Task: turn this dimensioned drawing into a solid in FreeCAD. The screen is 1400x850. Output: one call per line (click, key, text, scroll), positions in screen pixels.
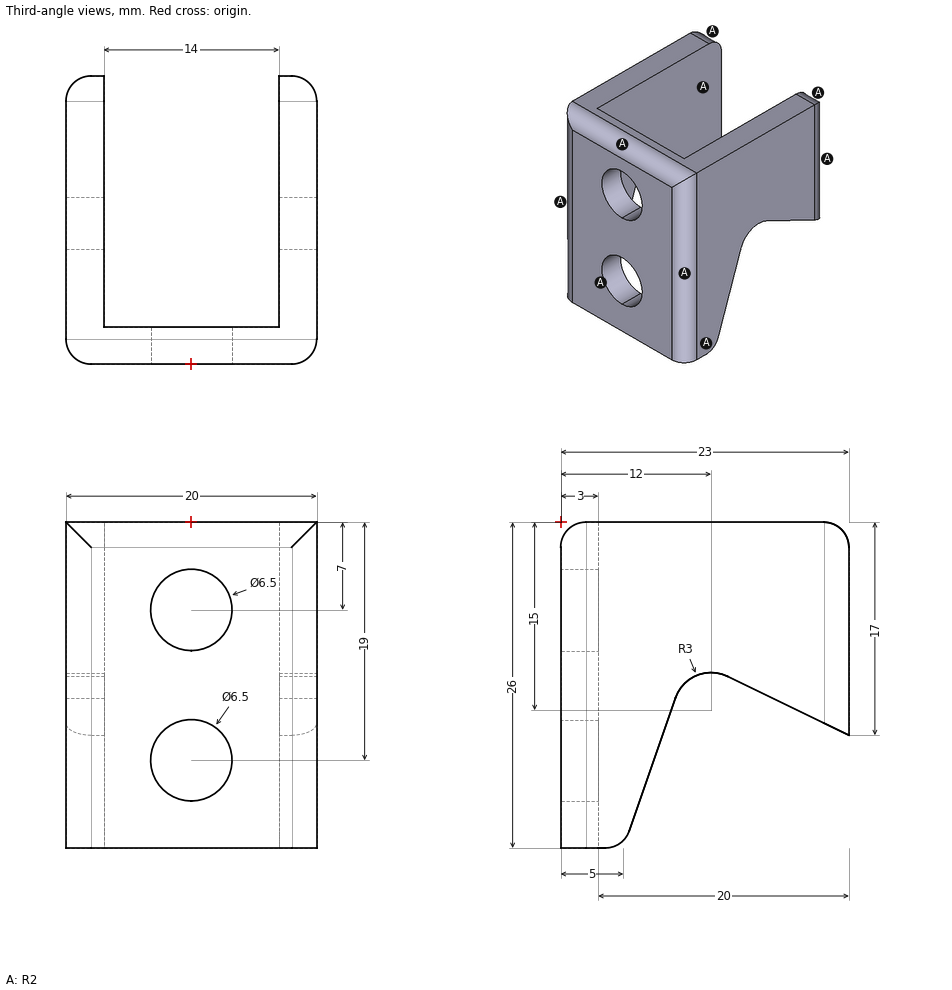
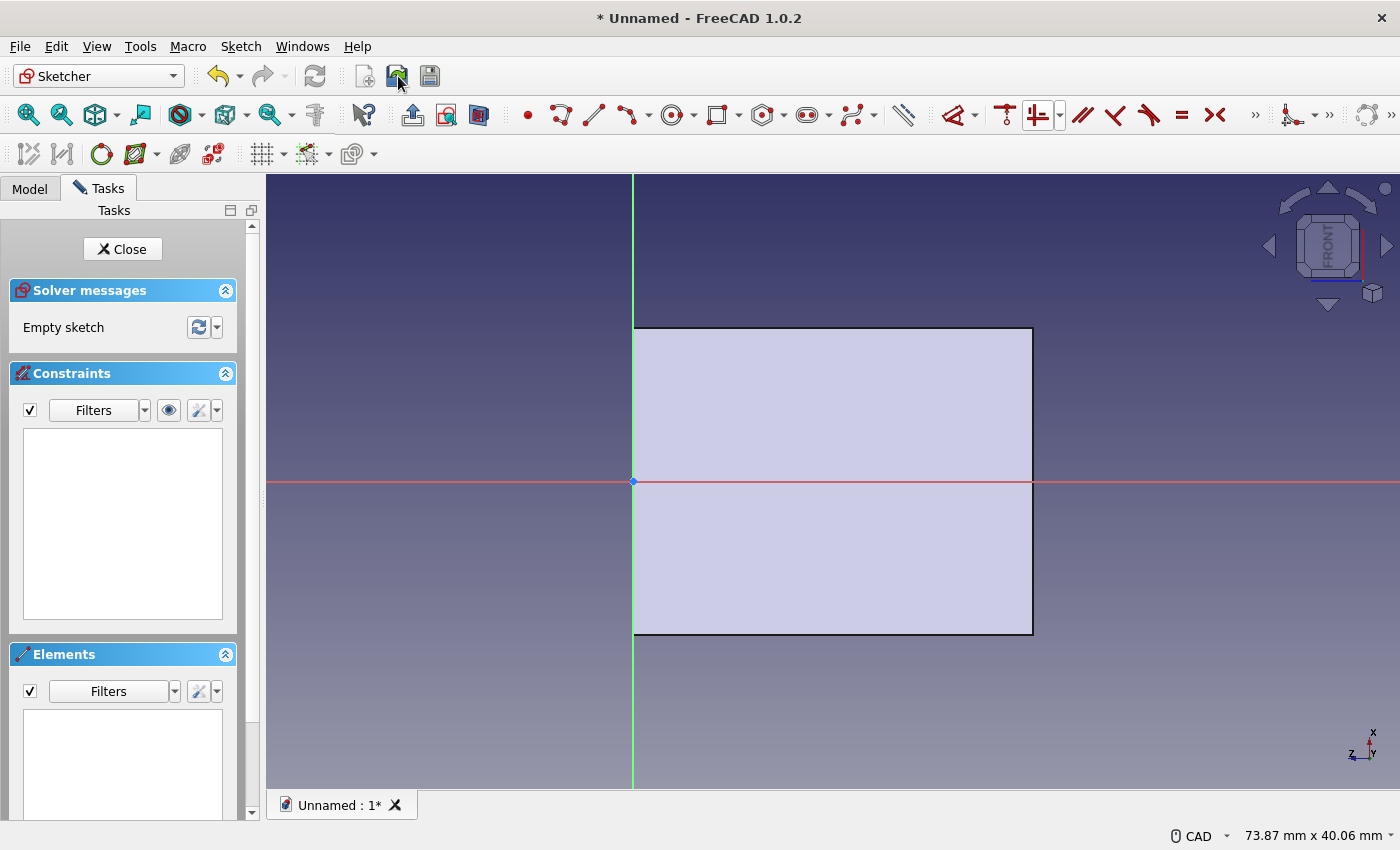
scroll(695, 481, up, 7)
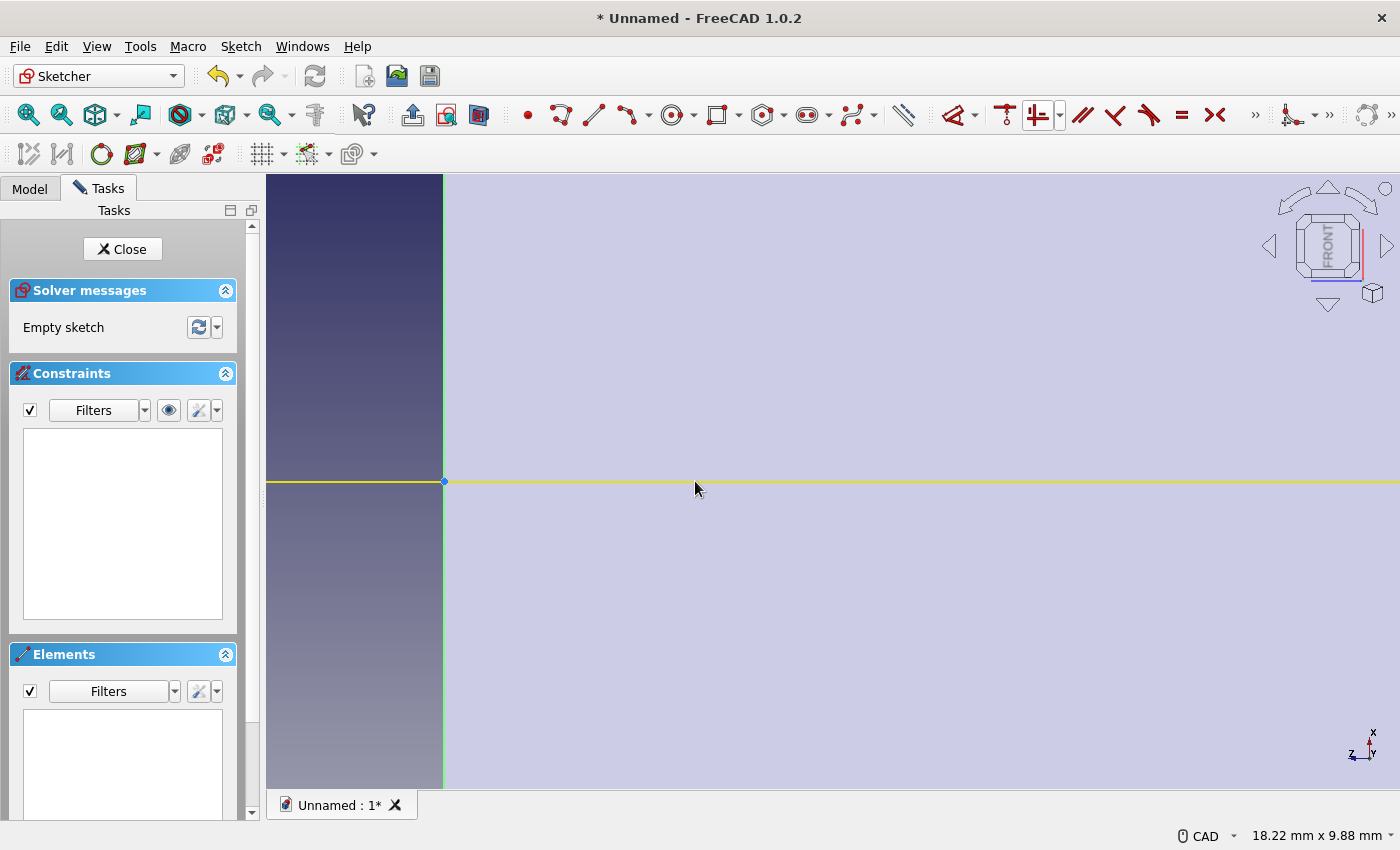
click(672, 116)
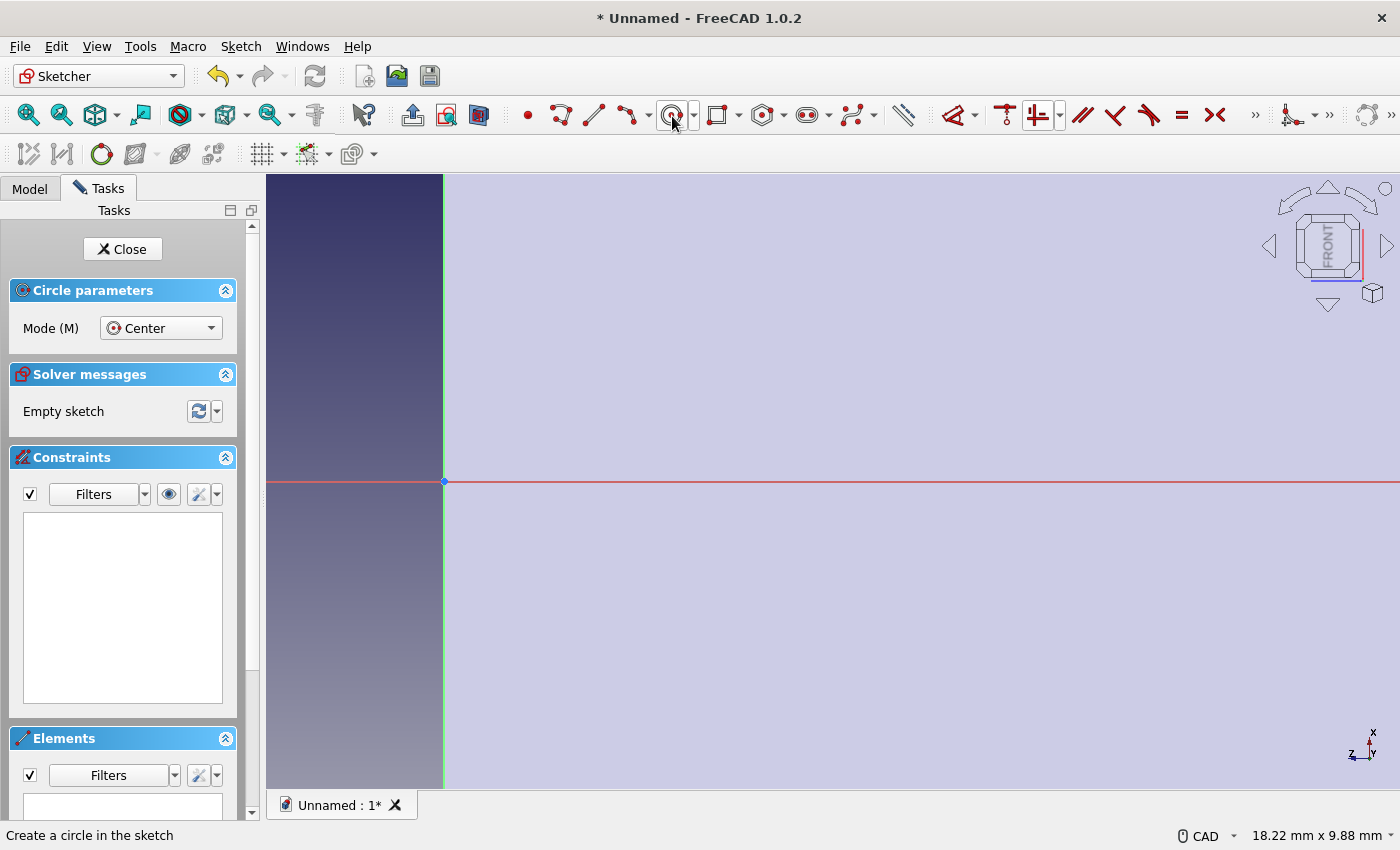
click(880, 482)
click(1023, 338)
key(Escape)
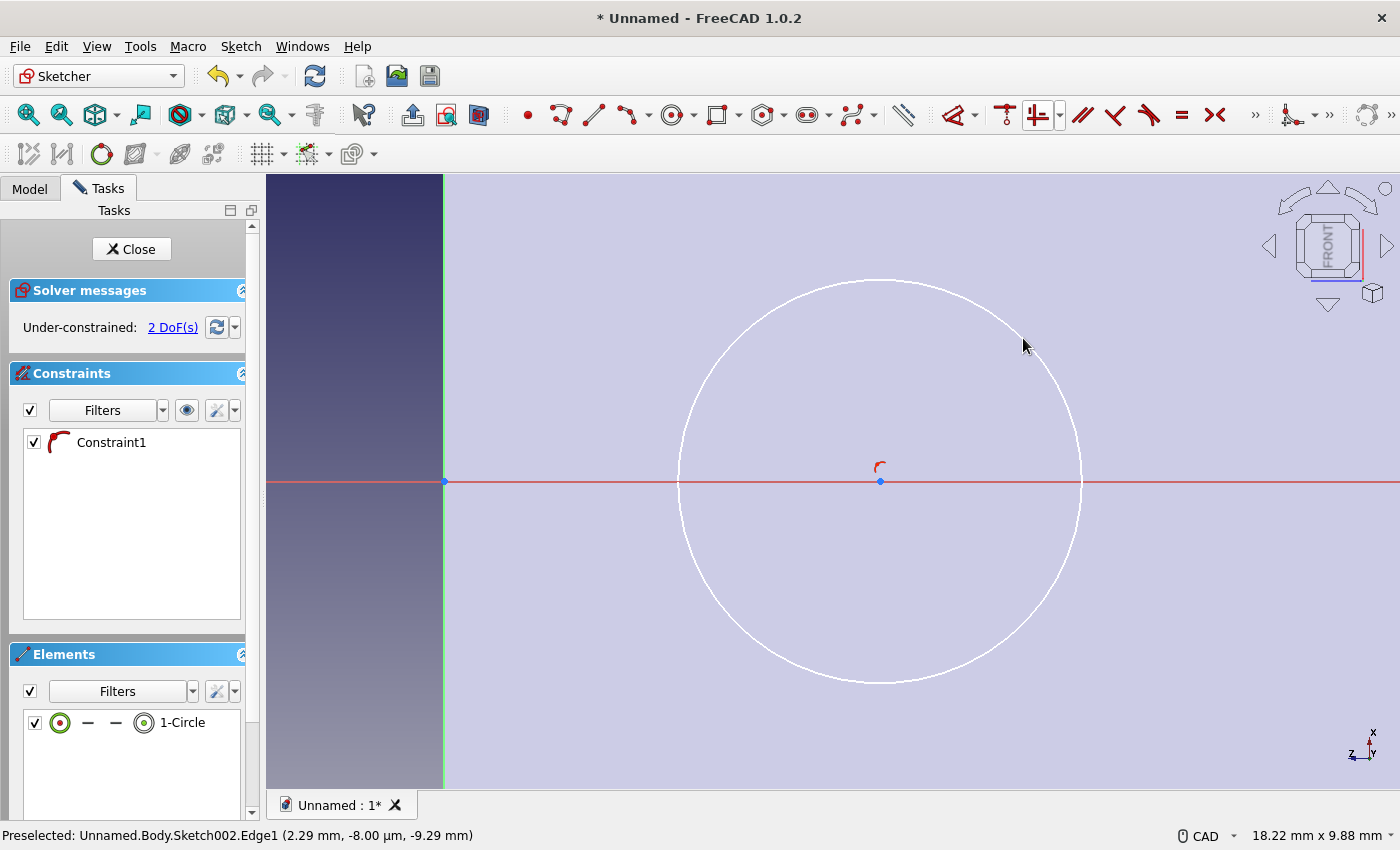
click(952, 116)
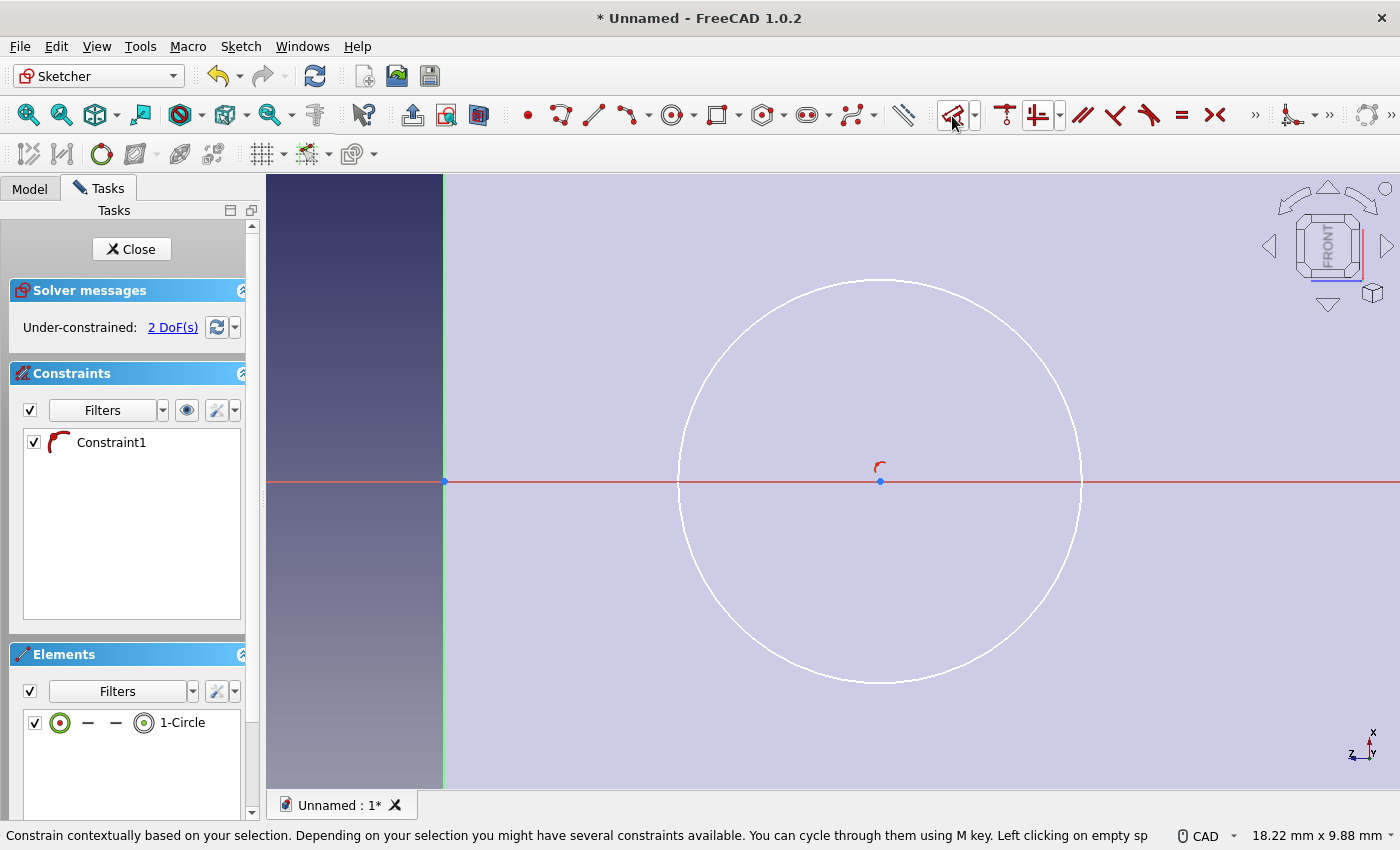
click(1022, 338)
click(1045, 315)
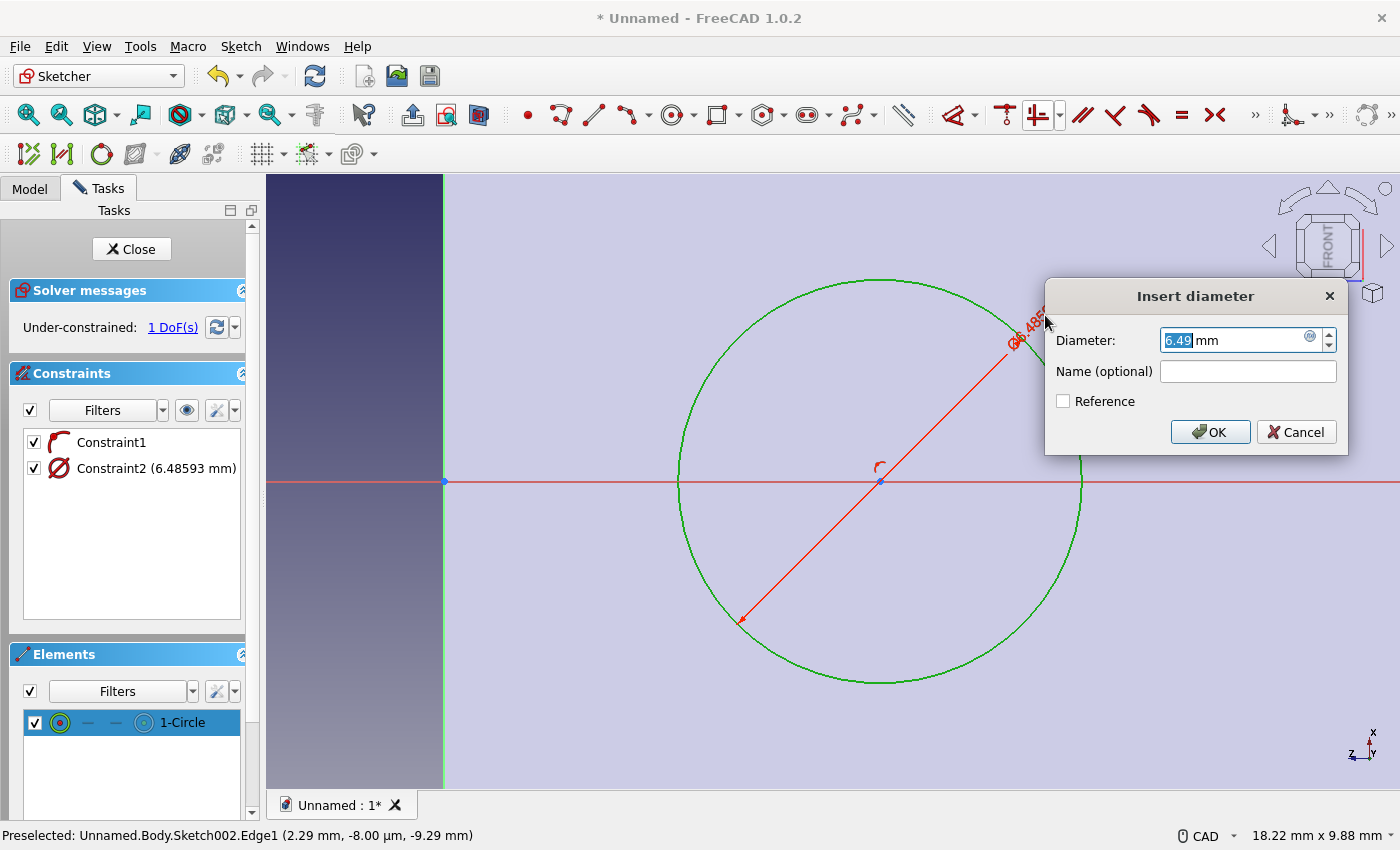
text(6.5)
key(Return)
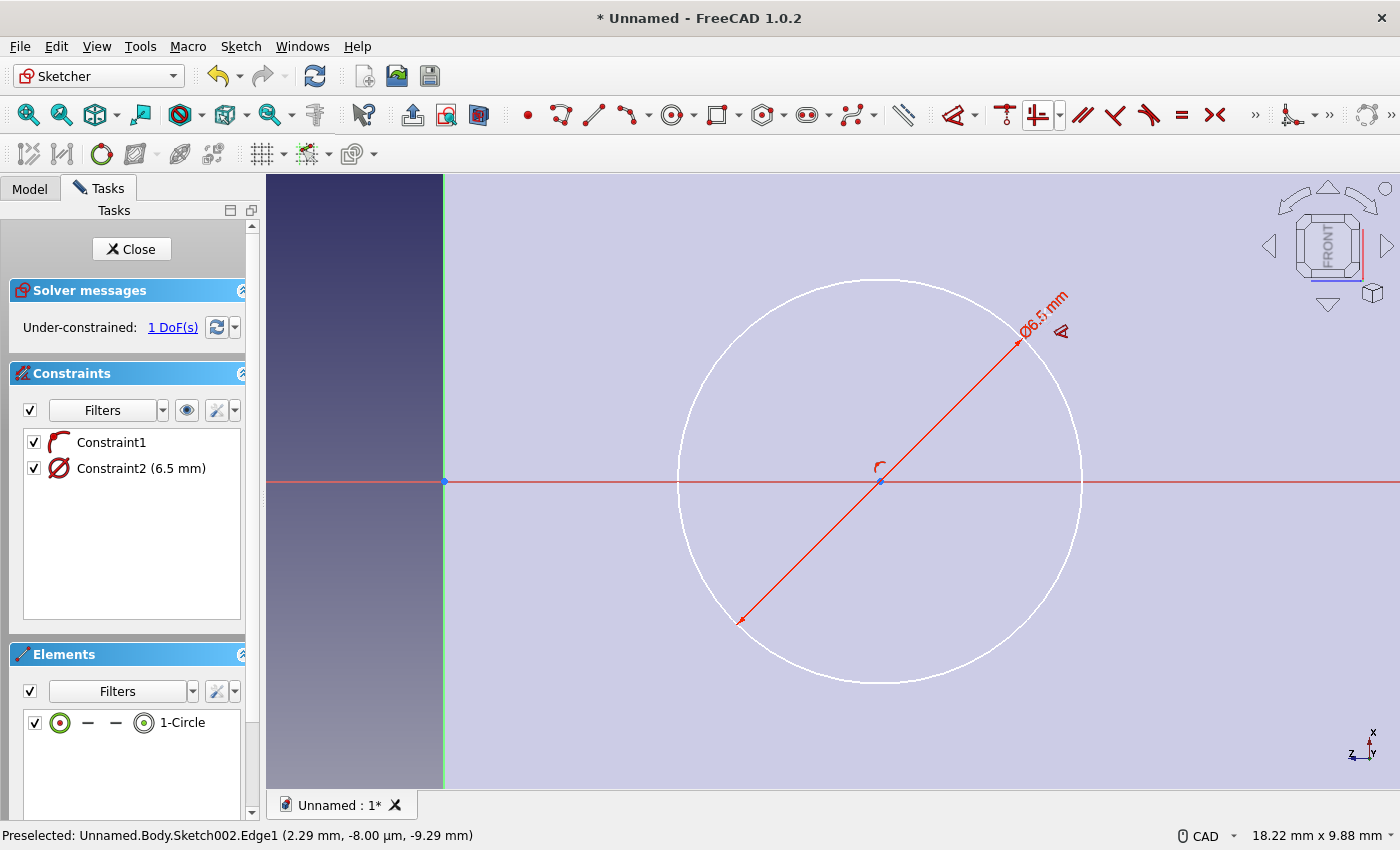
click(880, 482)
click(662, 516)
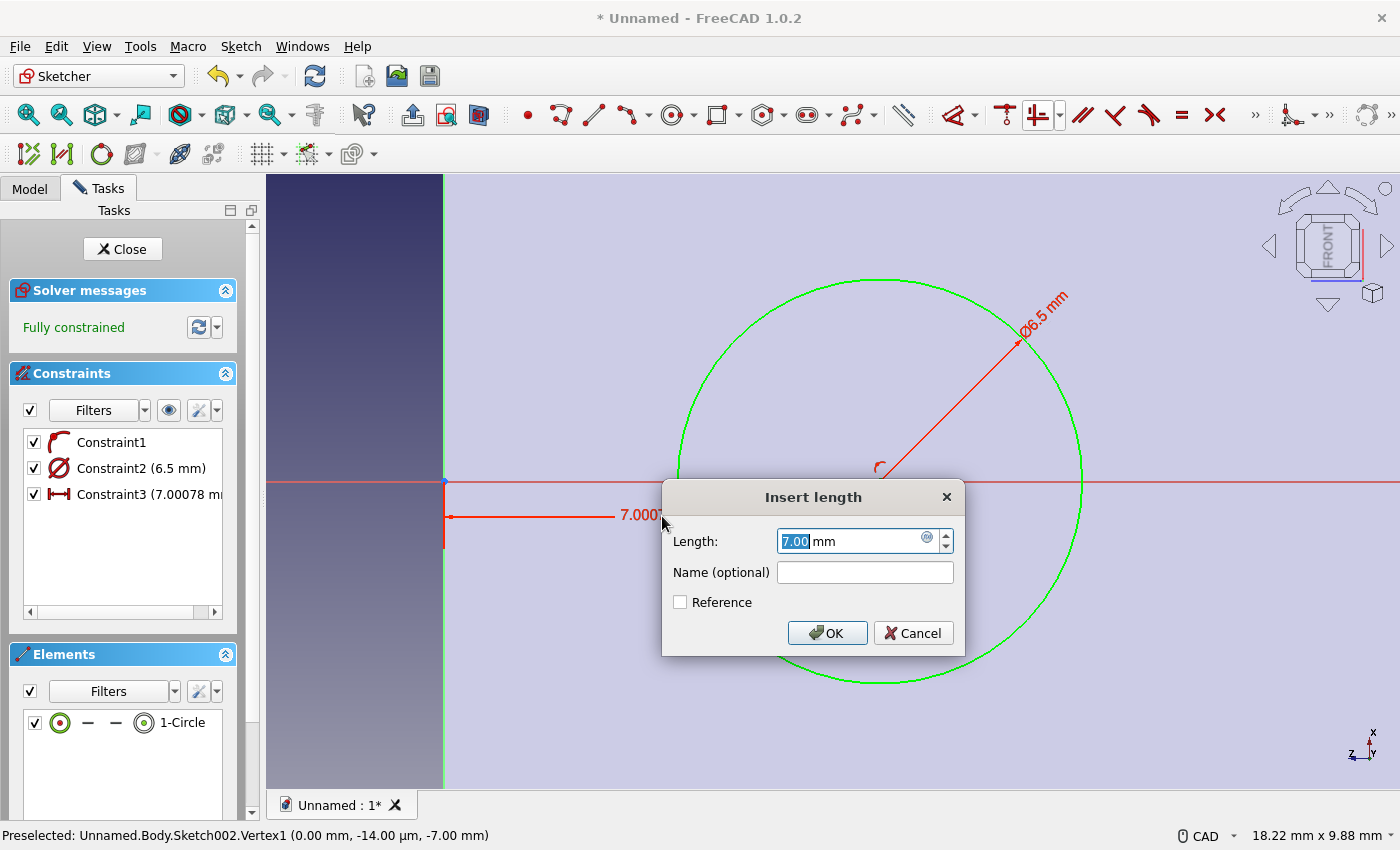
text(7)
key(Return)
key(Escape)